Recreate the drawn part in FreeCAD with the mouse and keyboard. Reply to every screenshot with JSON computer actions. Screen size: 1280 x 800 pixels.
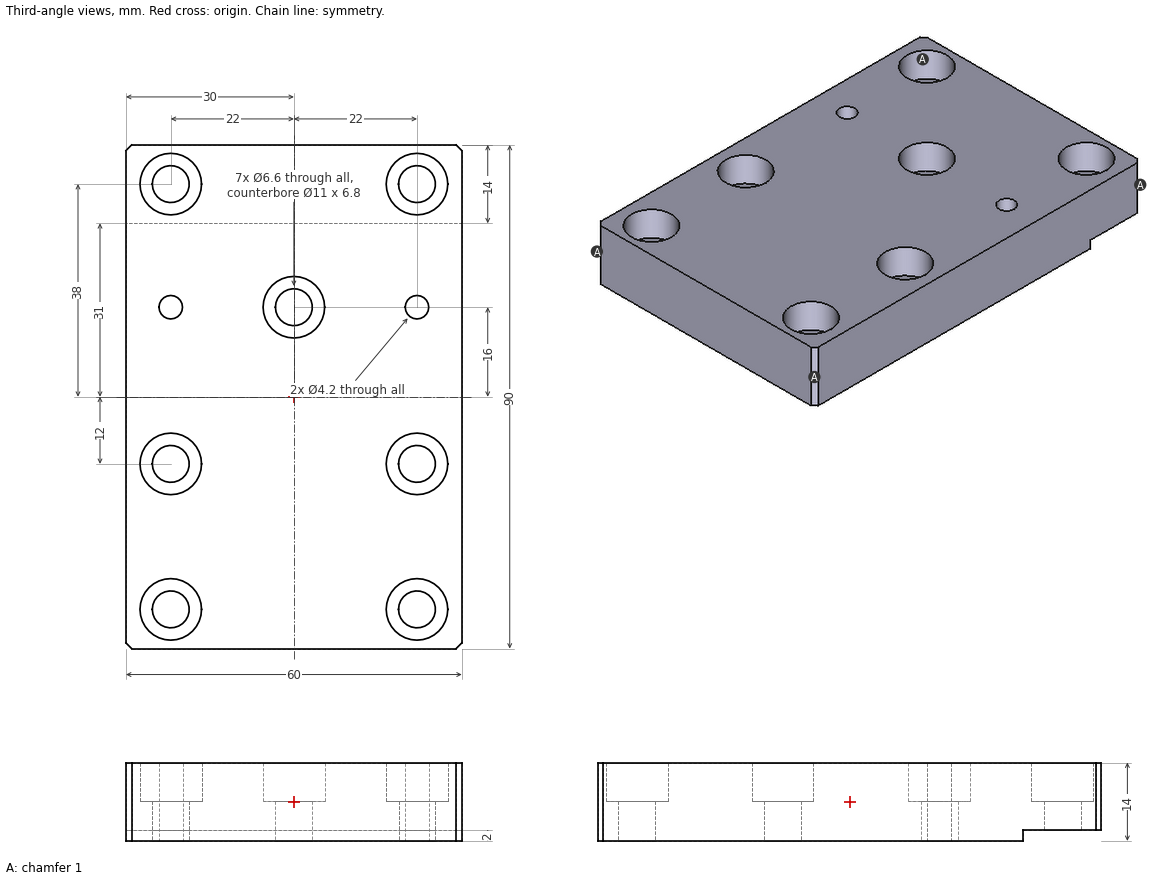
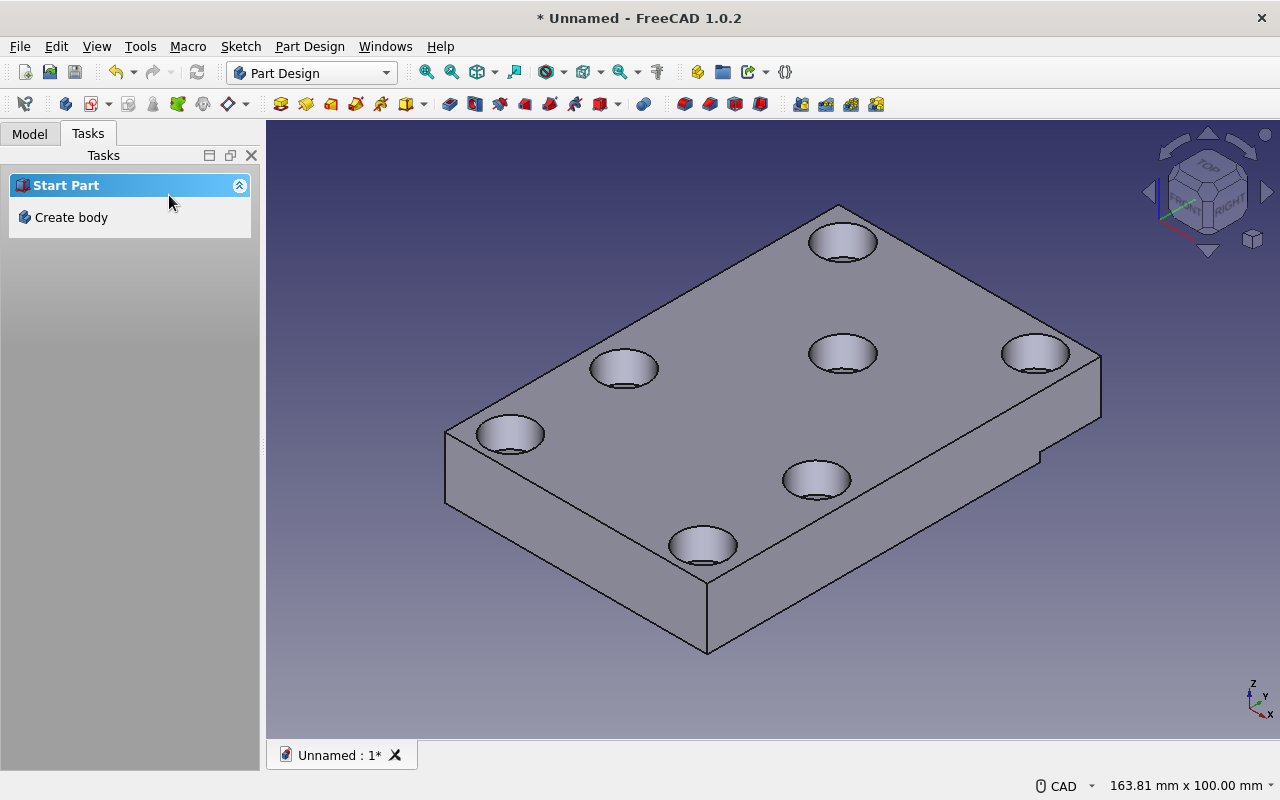
{"action": "left_click", "coordinate": [707, 618]}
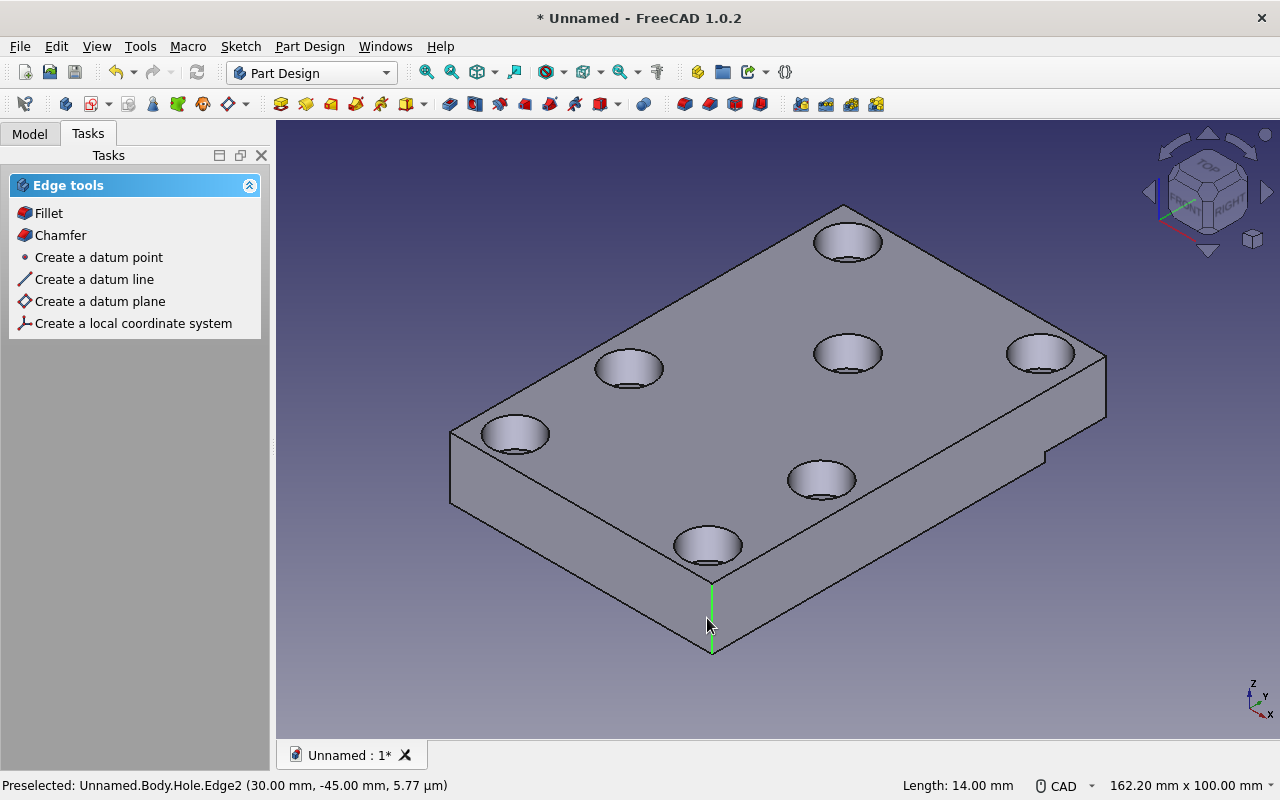
{"action": "key", "text": "2"}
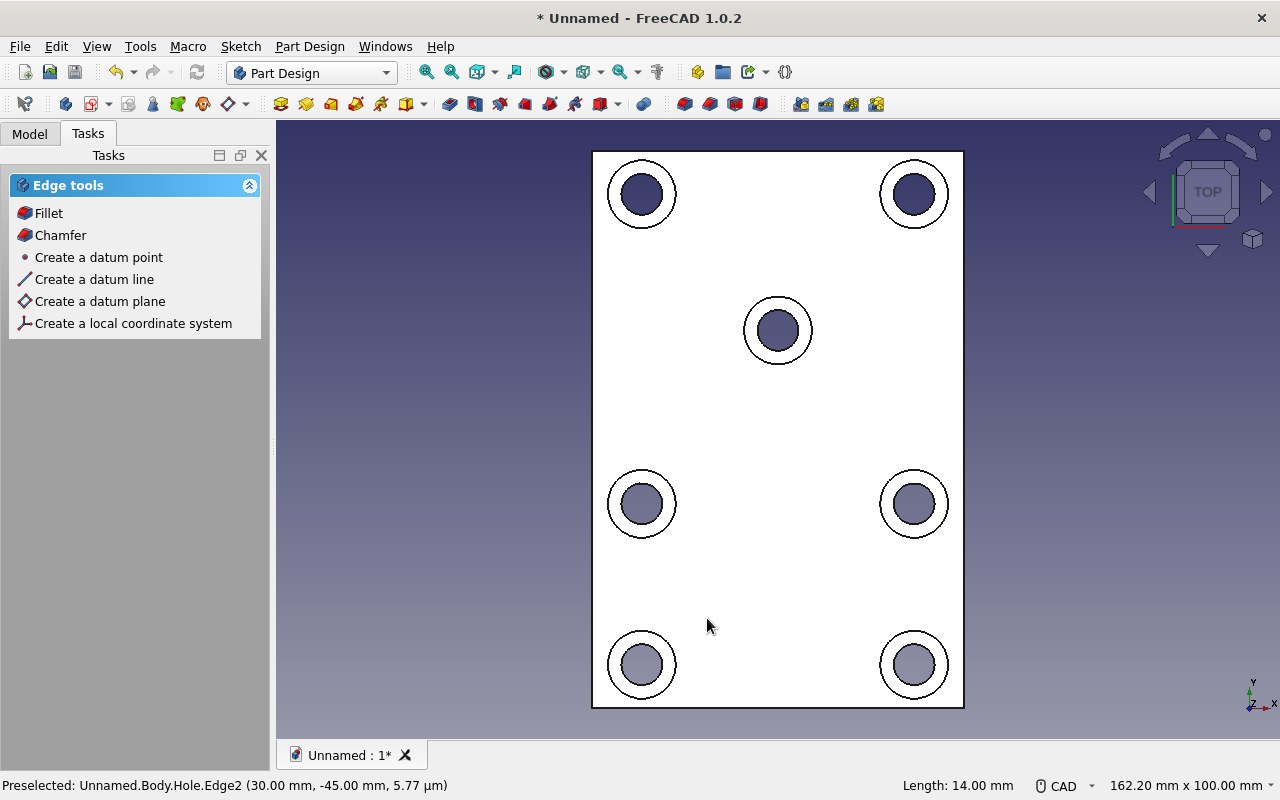
{"action": "key", "text": "0"}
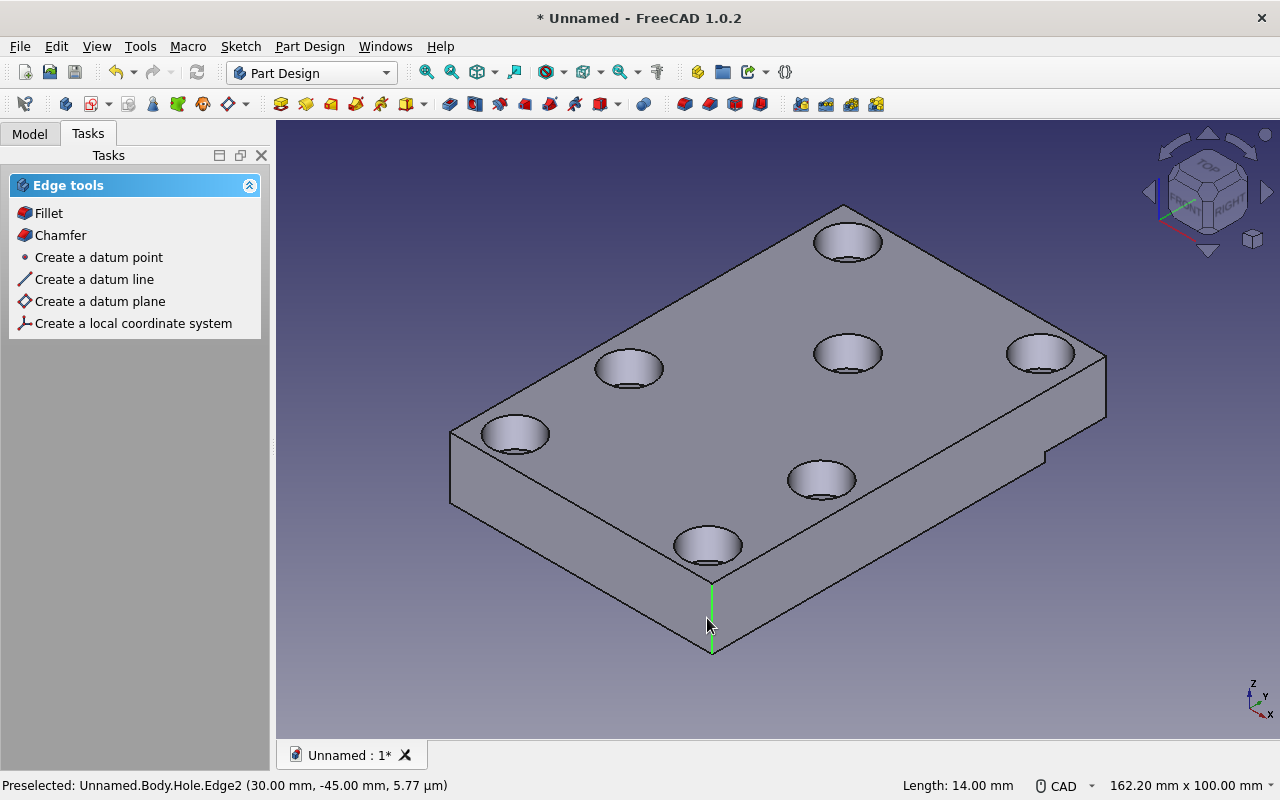
{"action": "key", "text": "1"}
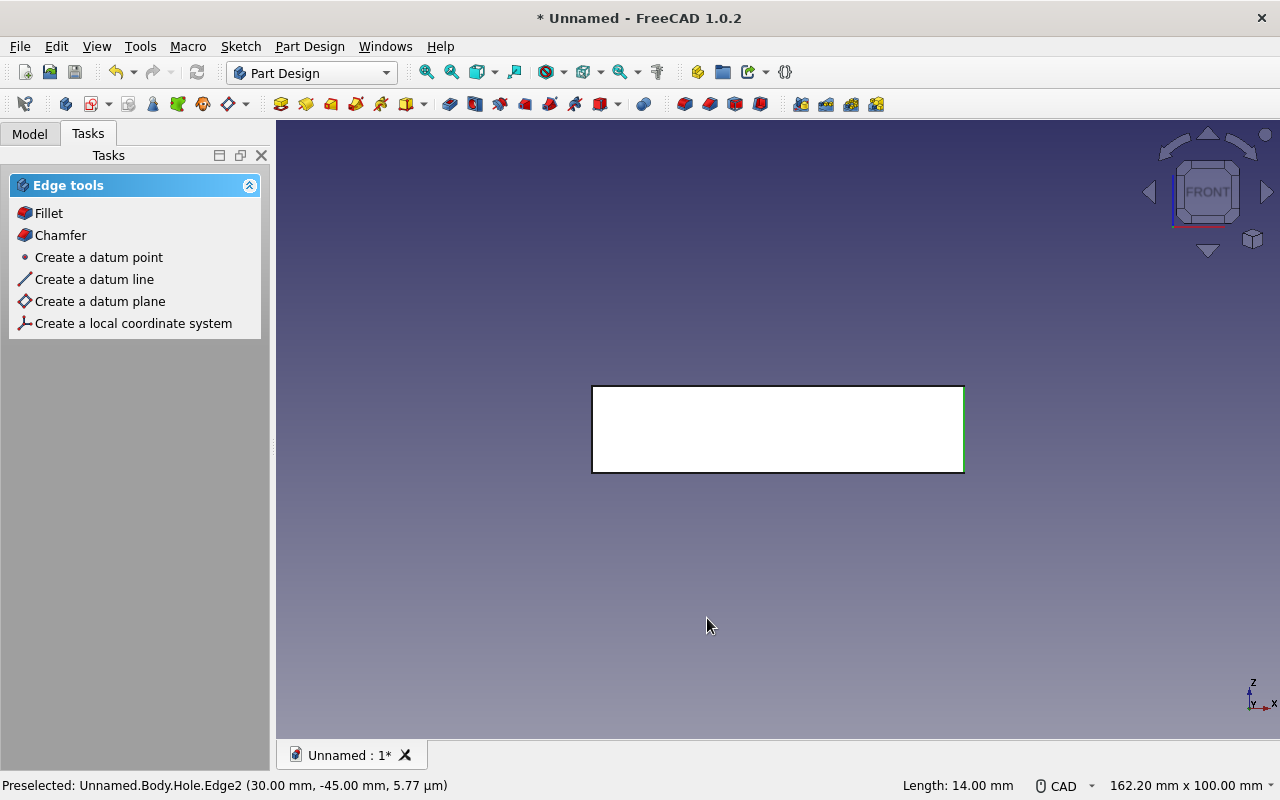
{"action": "left_click", "coordinate": [427, 72]}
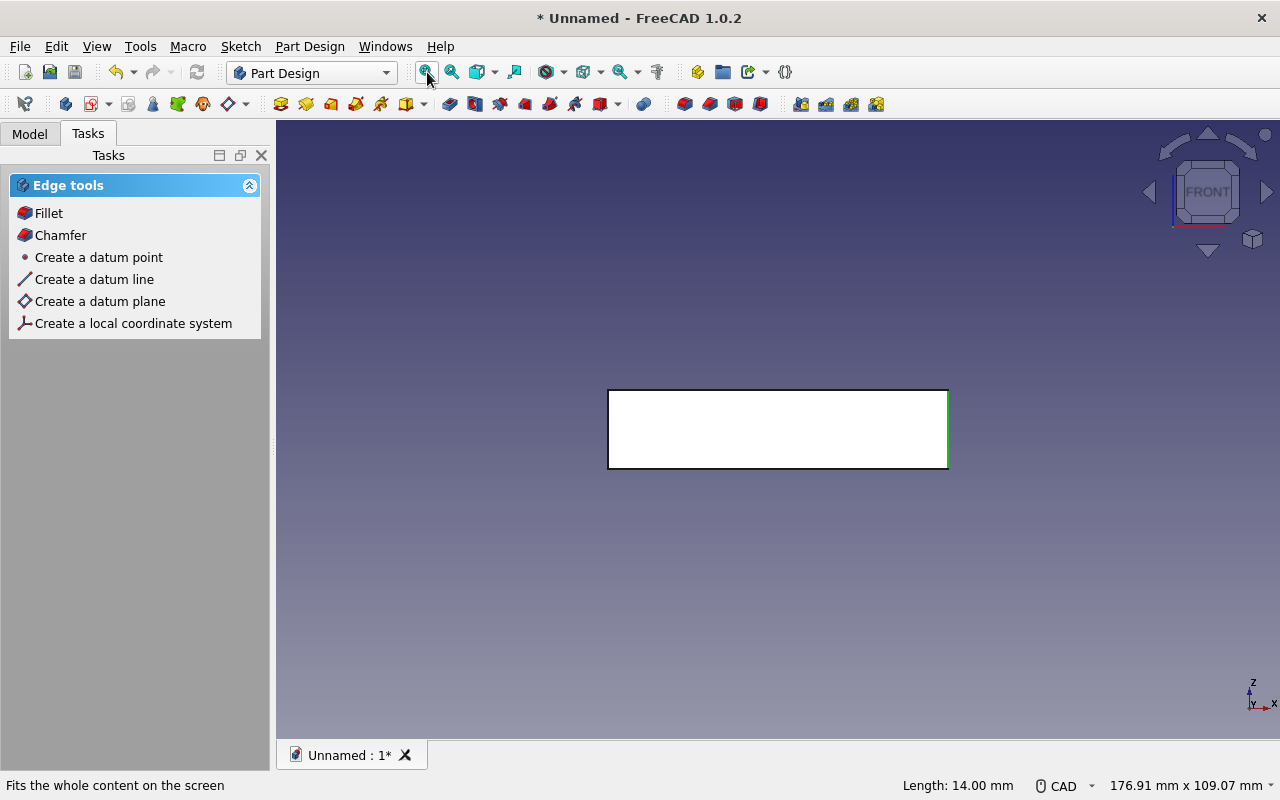
{"action": "left_click", "coordinate": [608, 429], "text": "ctrl"}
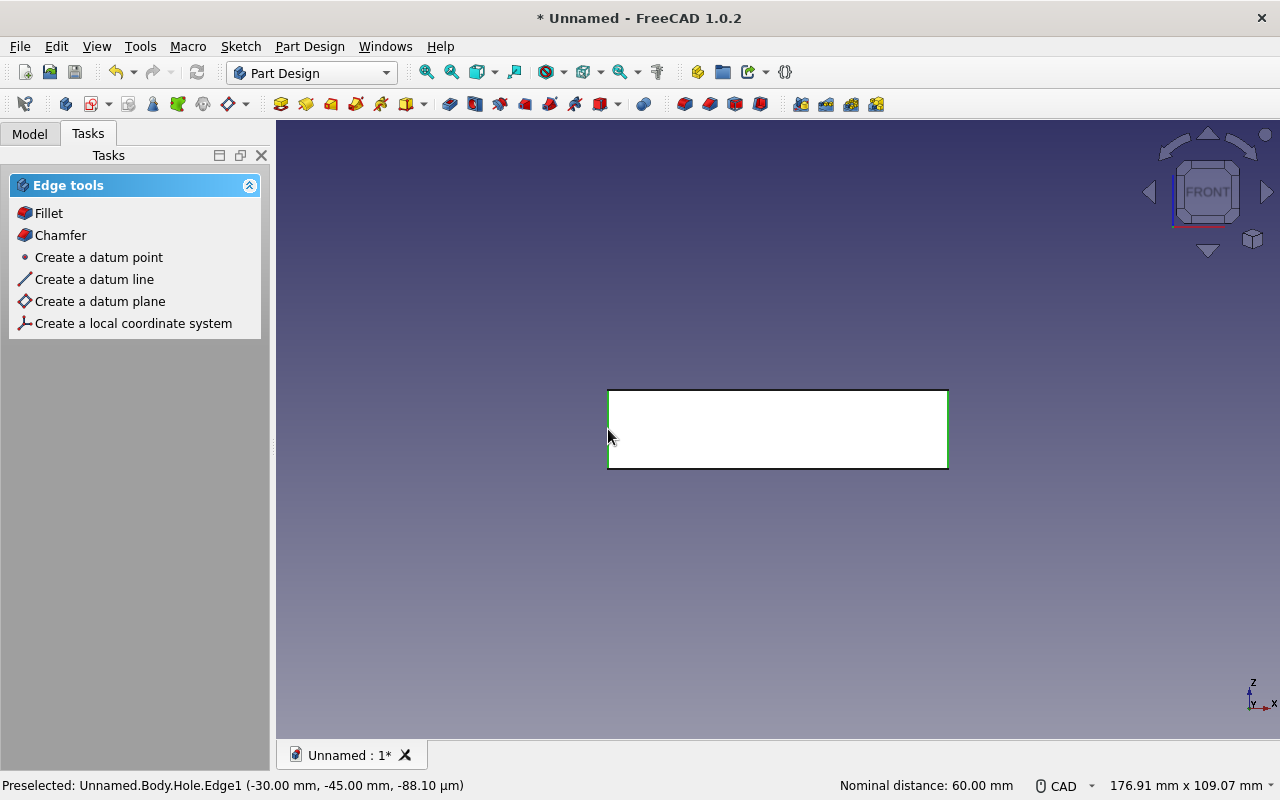
{"action": "key", "text": "3"}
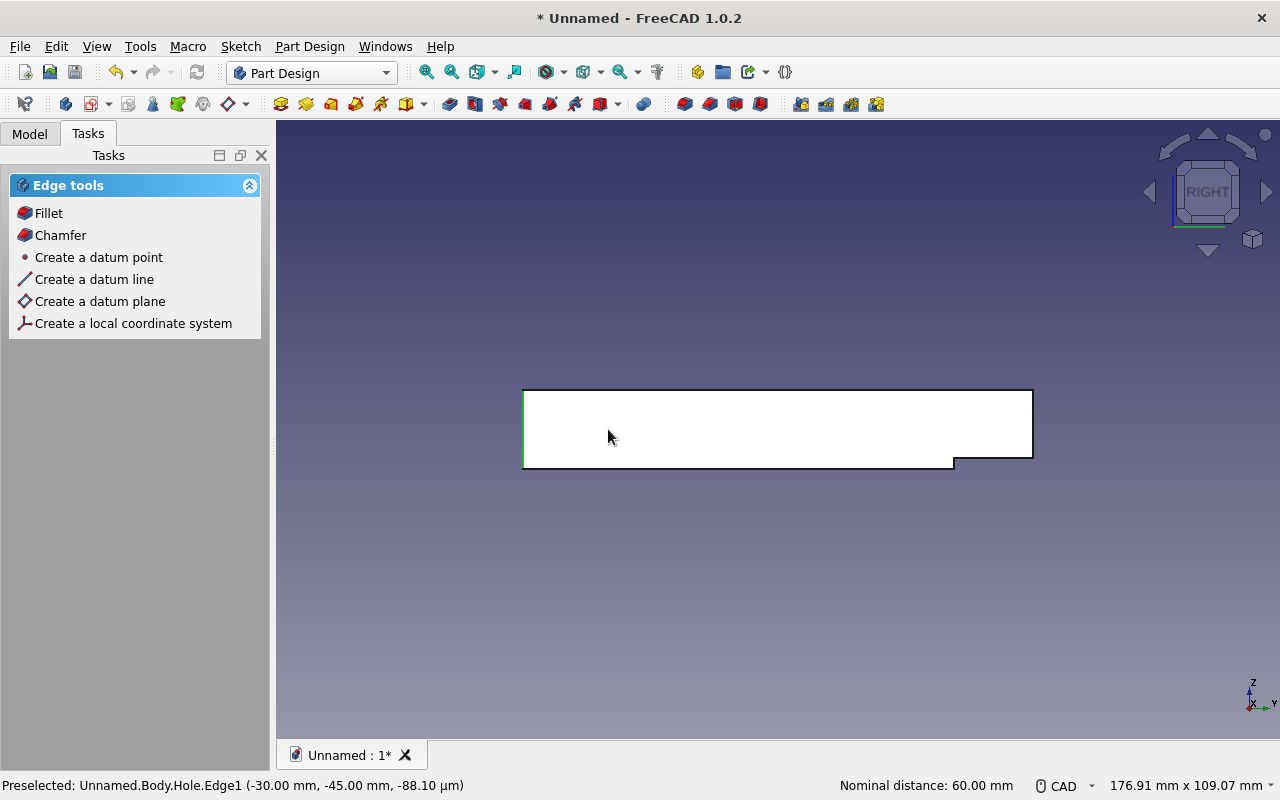
{"action": "left_click", "coordinate": [1033, 423], "text": "ctrl"}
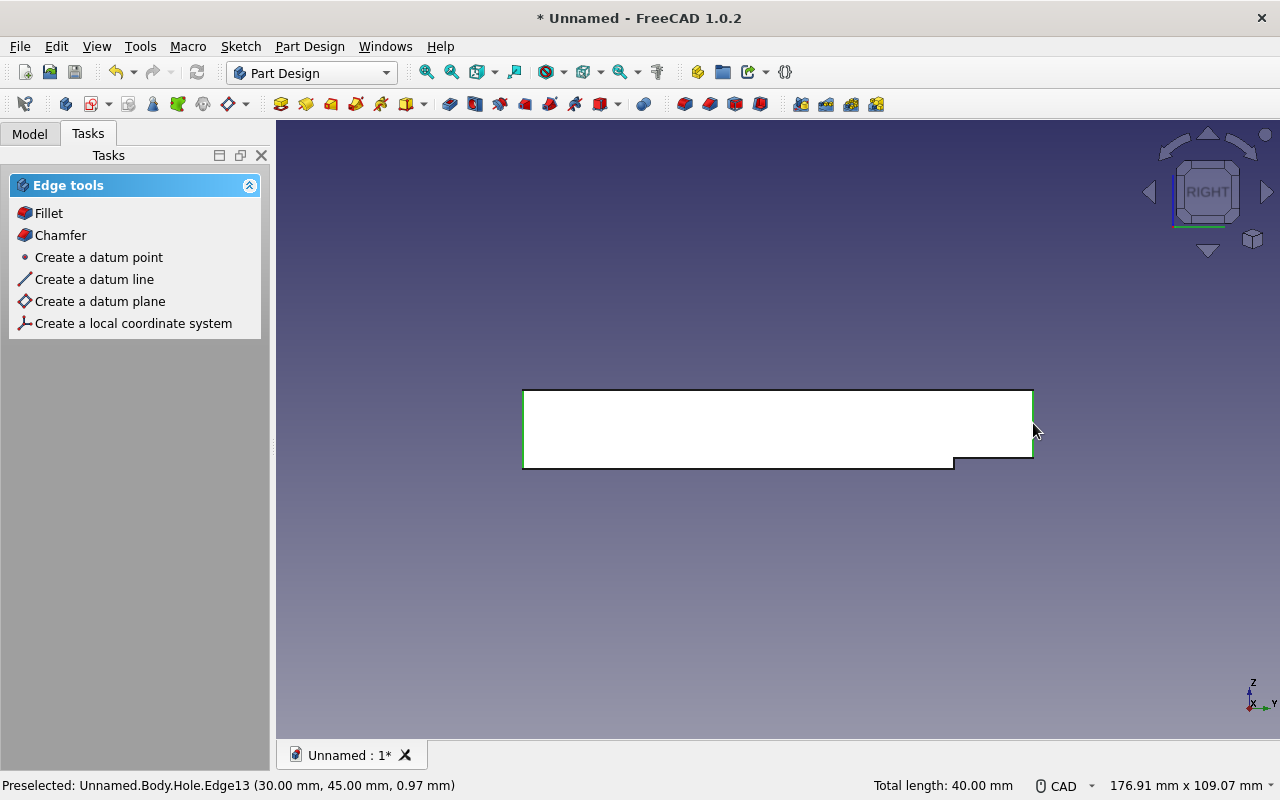
{"action": "key", "text": "5"}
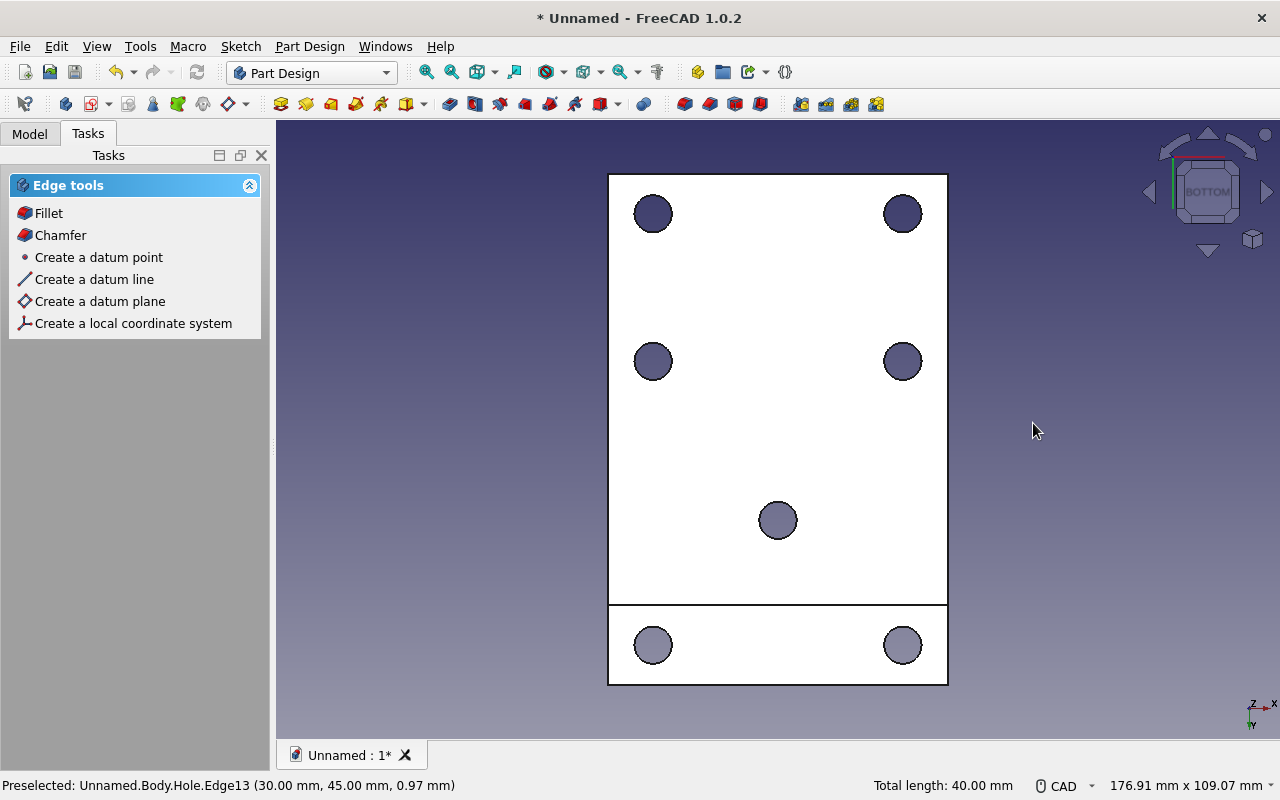
{"action": "key", "text": "4"}